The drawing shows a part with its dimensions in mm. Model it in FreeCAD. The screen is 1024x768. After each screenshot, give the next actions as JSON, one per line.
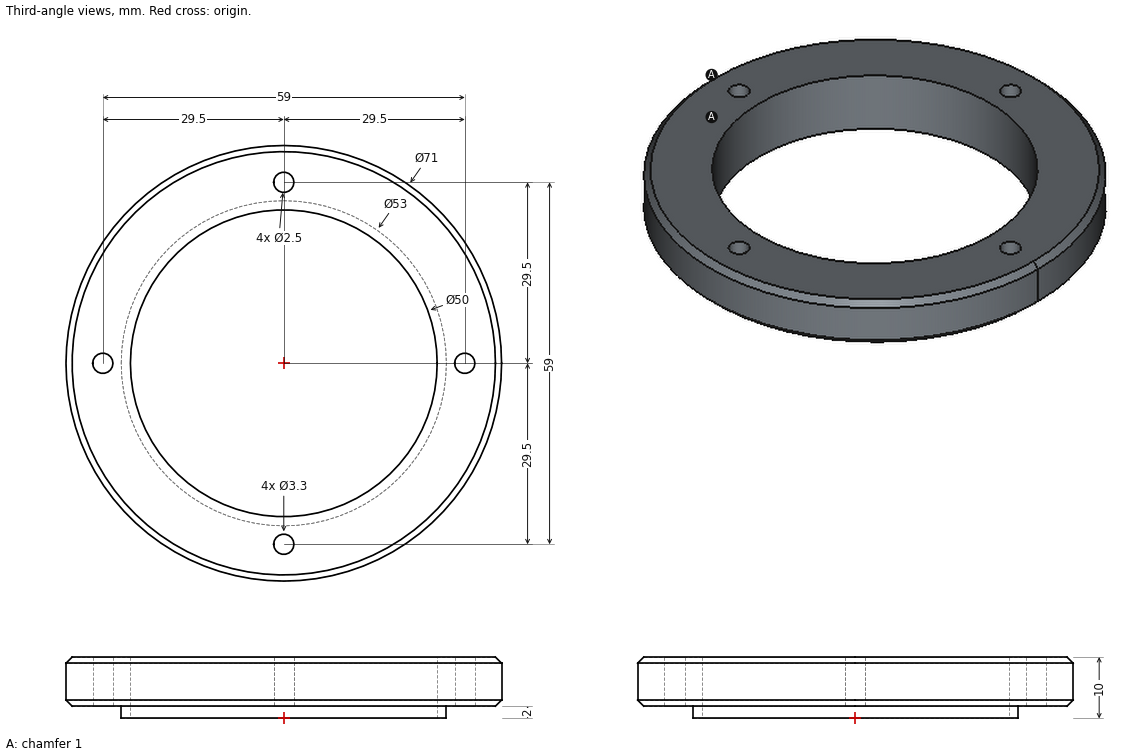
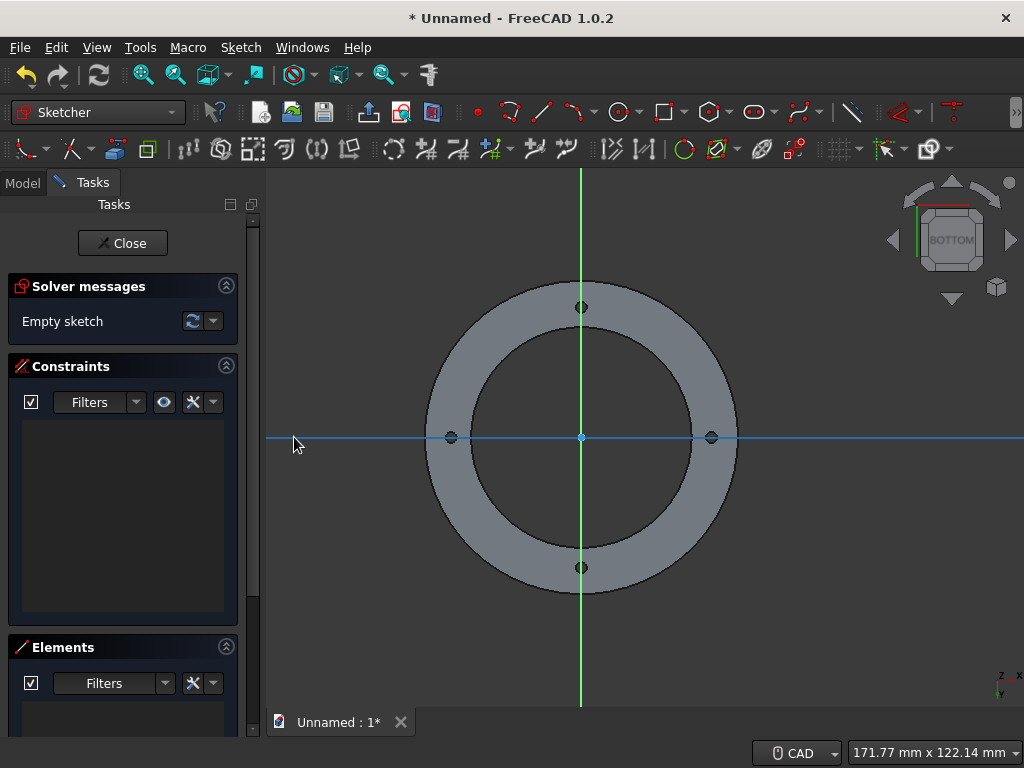
{"action": "key", "text": "g c"}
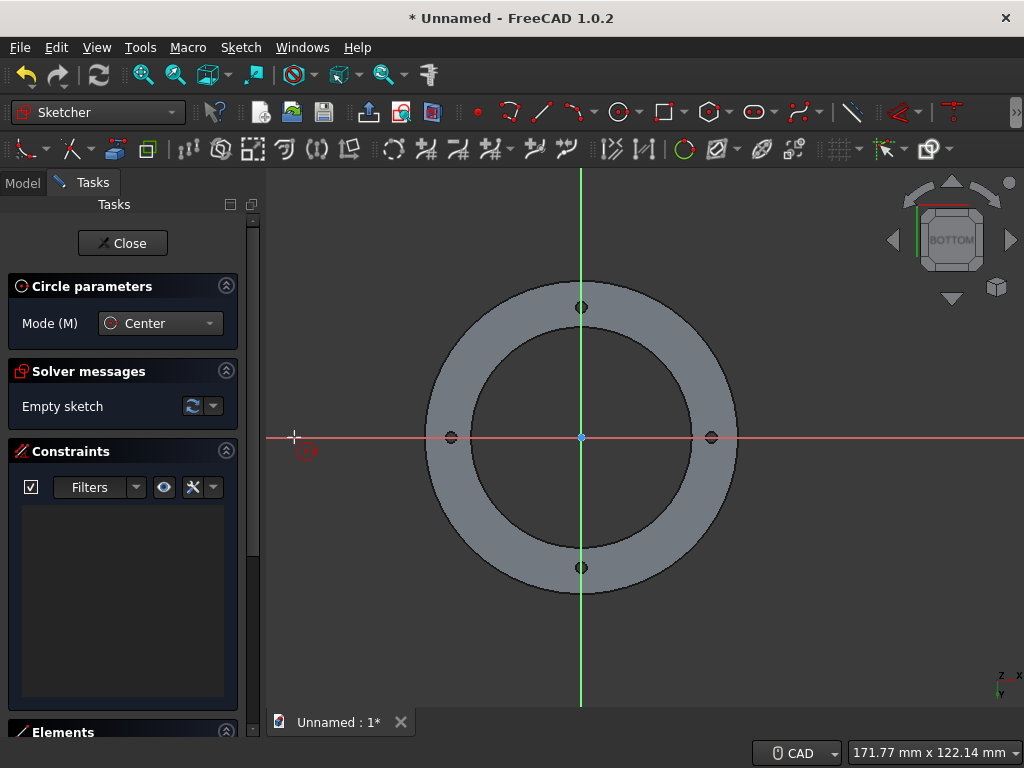
{"action": "left_click", "coordinate": [581, 438]}
{"action": "mouse_move", "coordinate": [692, 327]}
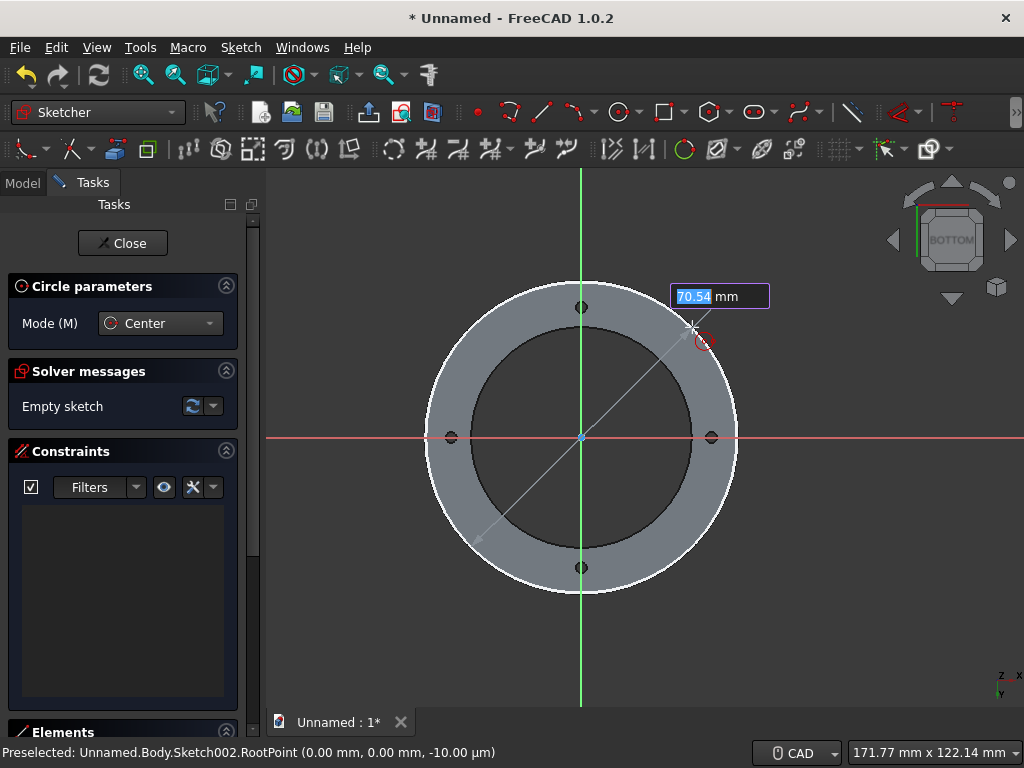
{"action": "type", "text": "71"}
{"action": "key", "text": "Return"}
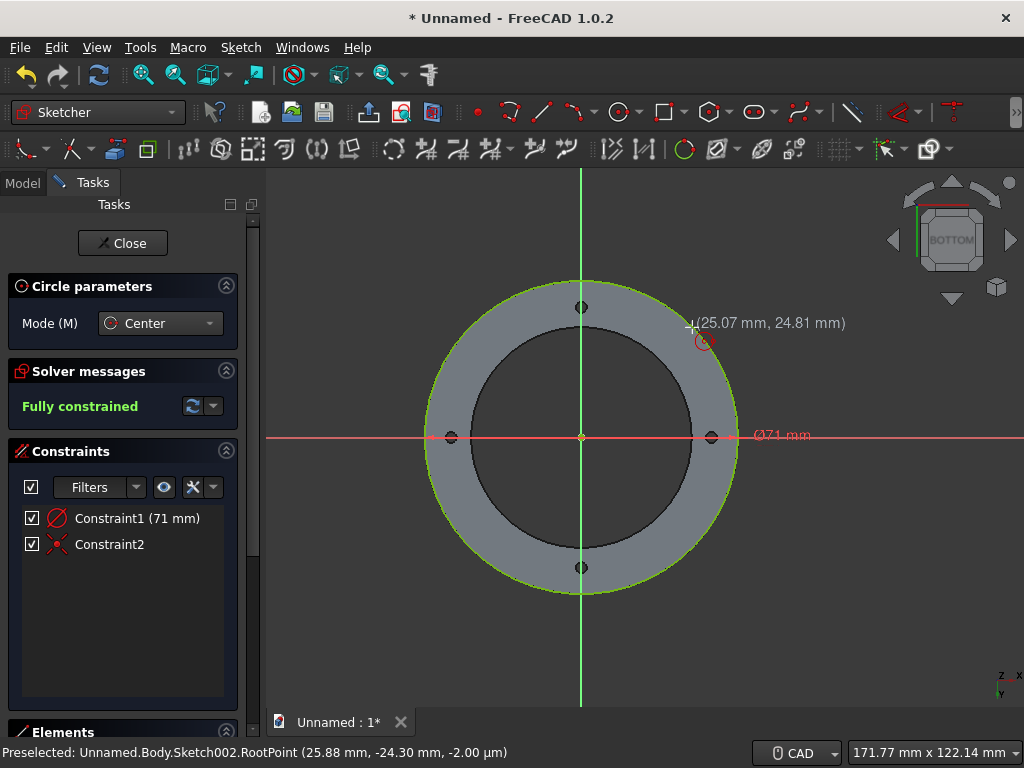
{"action": "left_click", "coordinate": [581, 438]}
{"action": "mouse_move", "coordinate": [664, 355]}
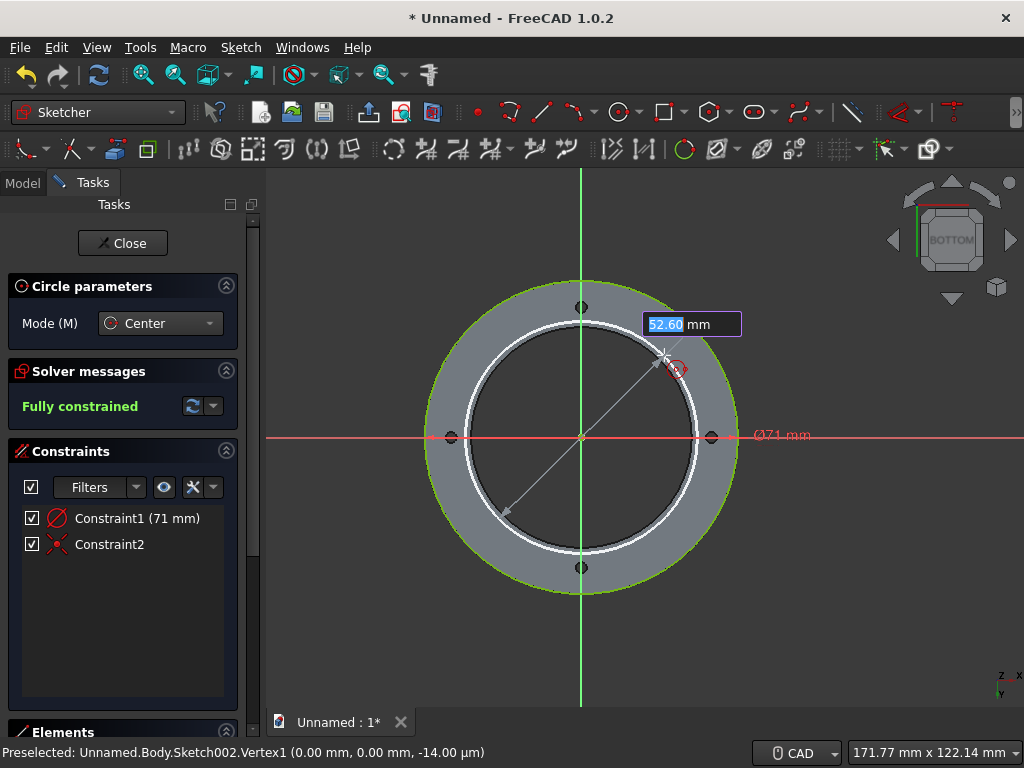
{"action": "type", "text": "53"}
{"action": "key", "text": "Return"}
{"action": "key", "text": "Escape"}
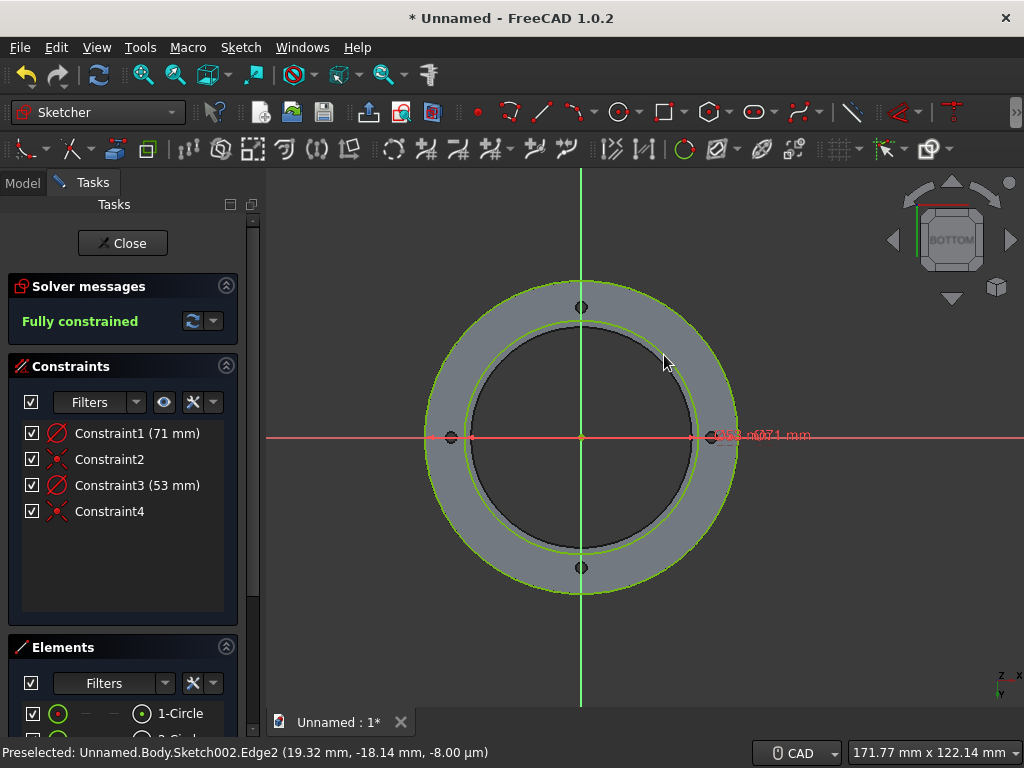
{"action": "left_click", "coordinate": [123, 243]}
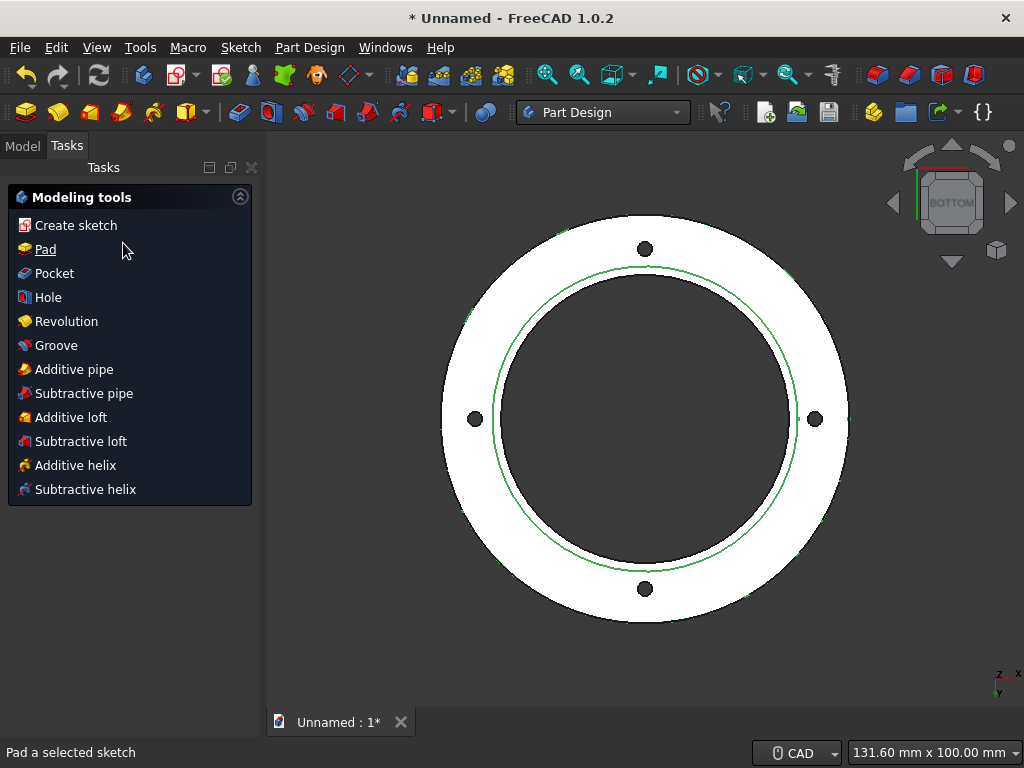
{"action": "left_click", "coordinate": [240, 112]}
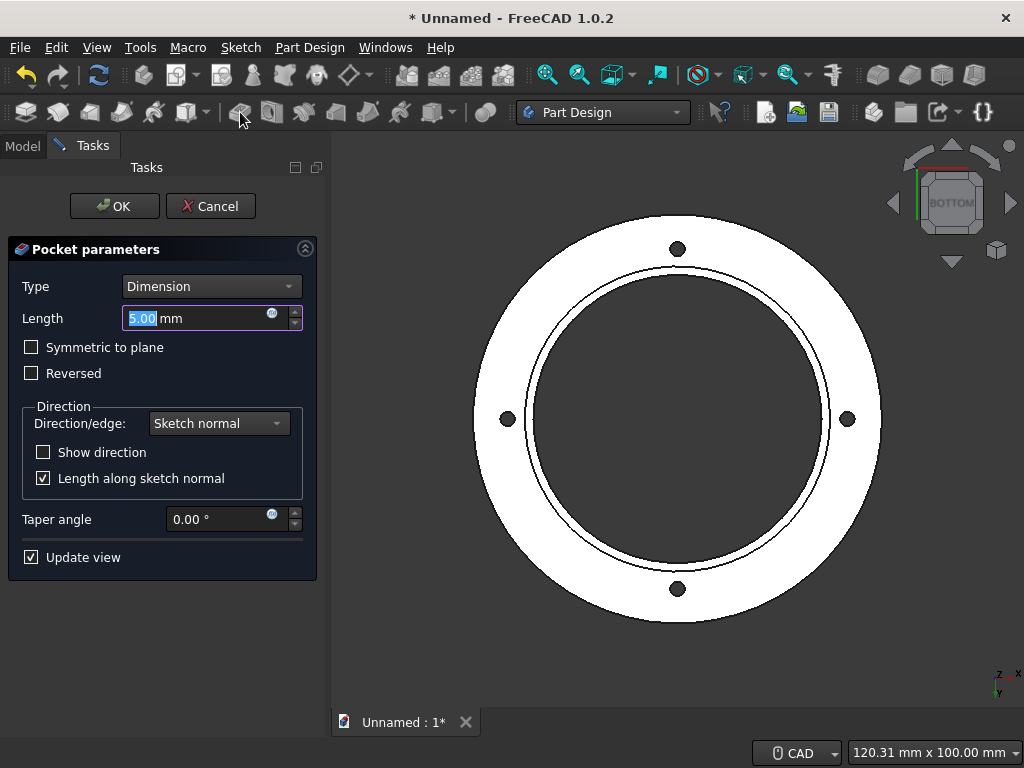
{"action": "type", "text": "2"}
{"action": "key", "text": "Tab"}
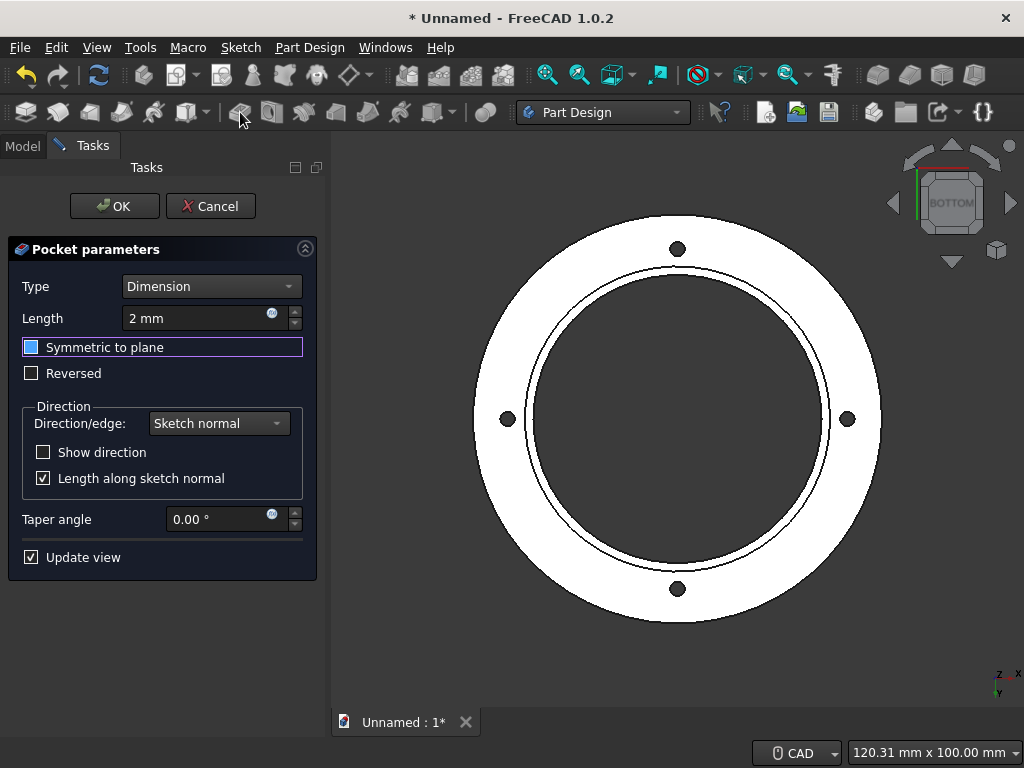
{"action": "left_click", "coordinate": [115, 206]}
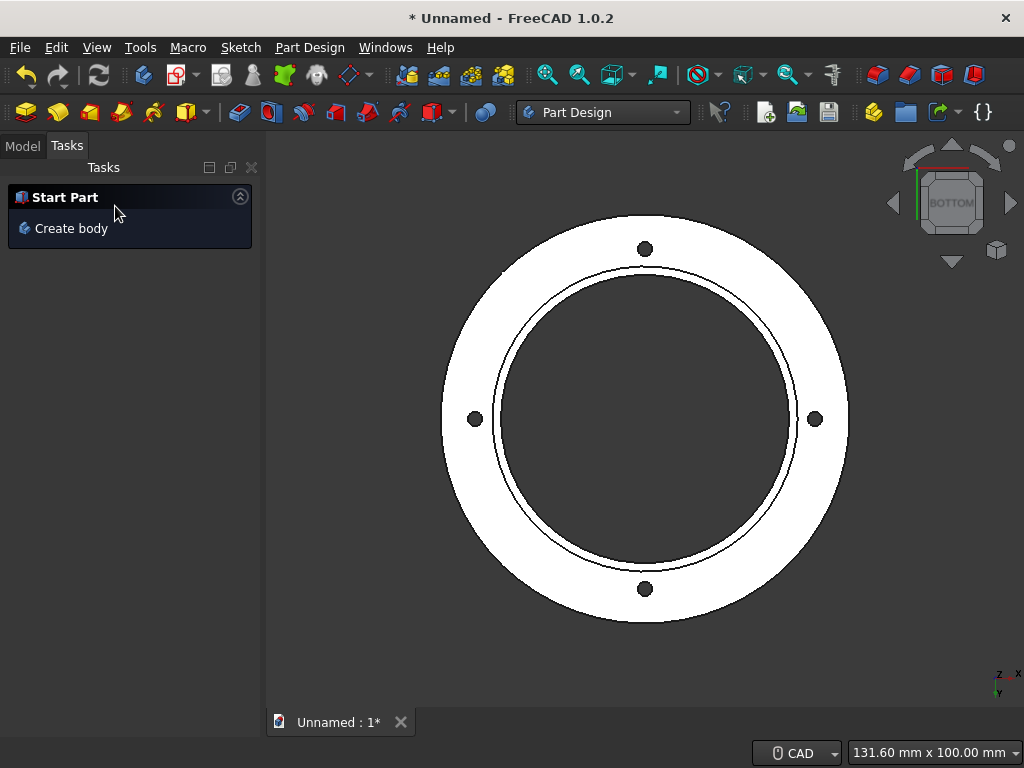
{"action": "key", "text": "0"}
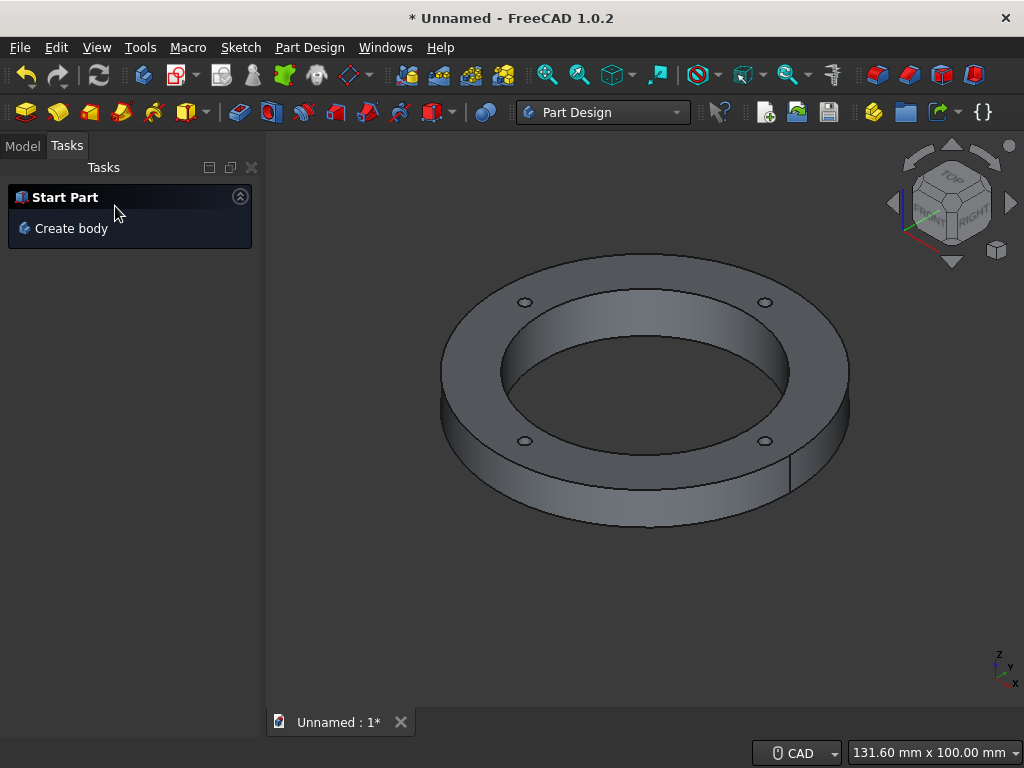
{"action": "left_click", "coordinate": [810, 371]}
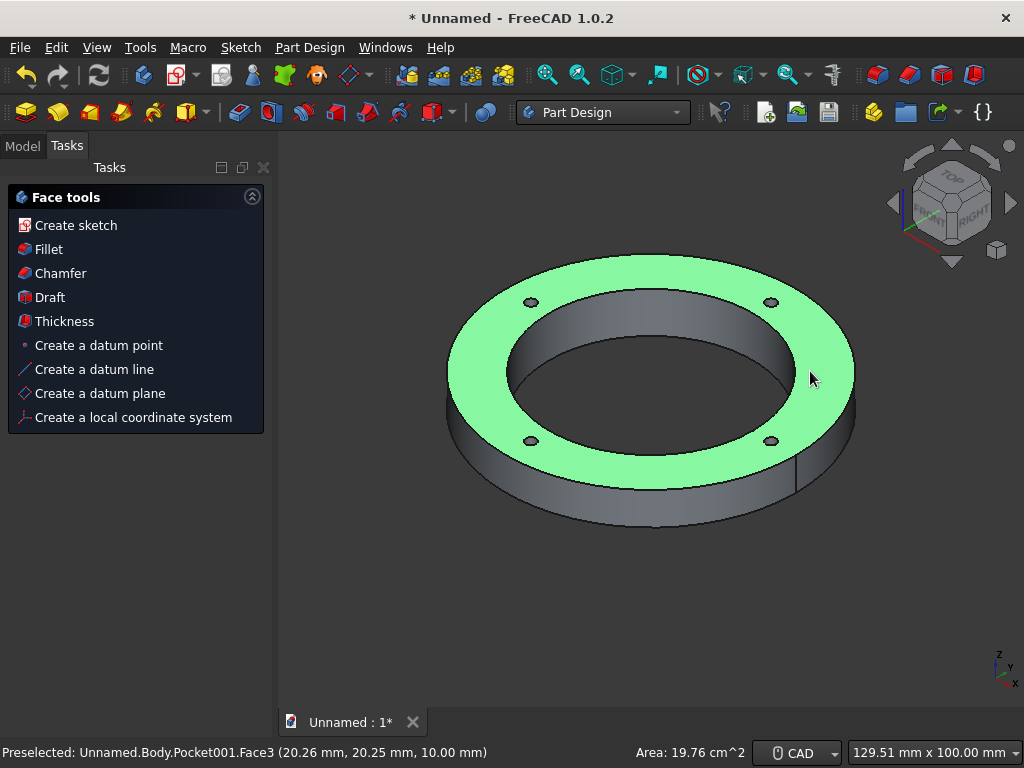
{"action": "left_click", "coordinate": [176, 76]}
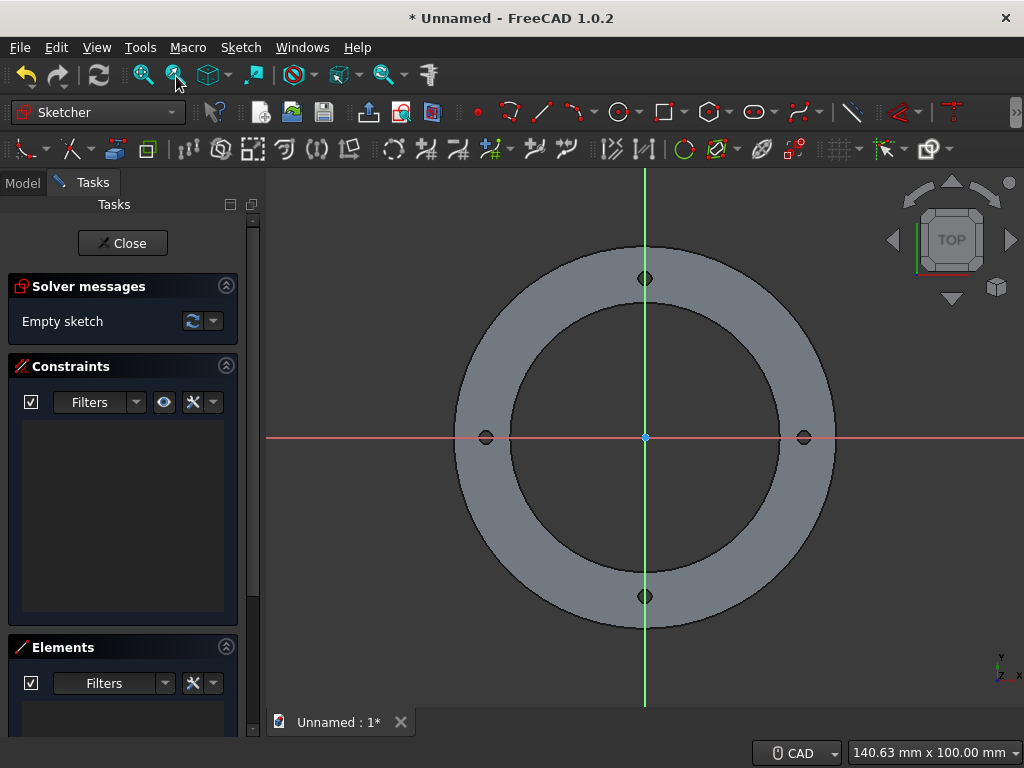
{"action": "left_click", "coordinate": [620, 112]}